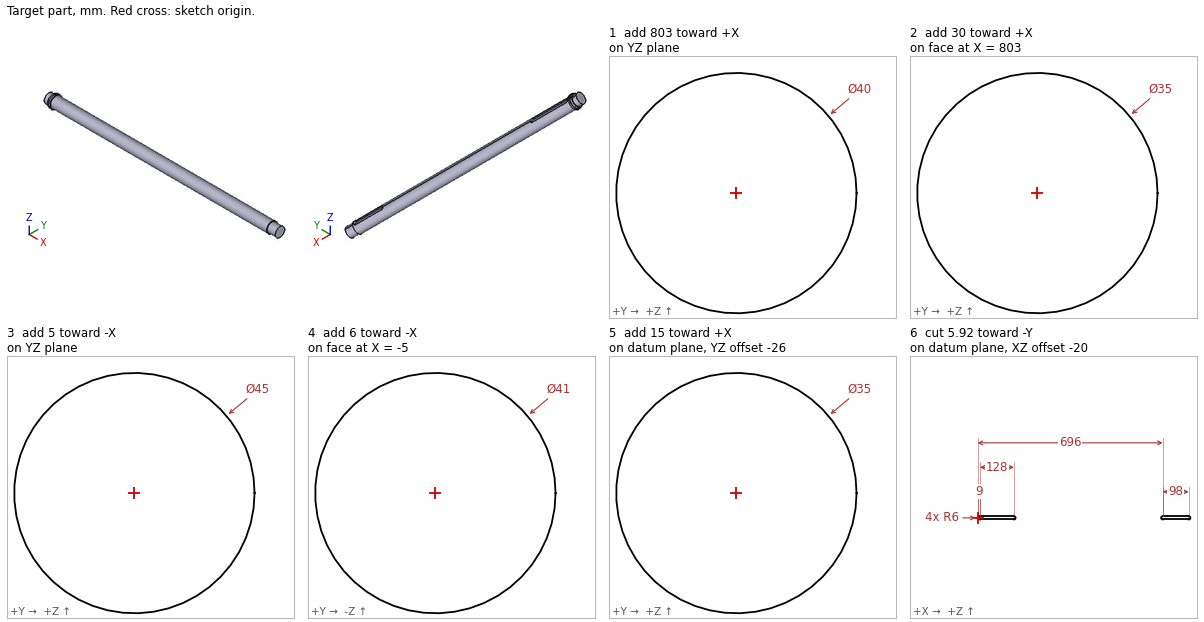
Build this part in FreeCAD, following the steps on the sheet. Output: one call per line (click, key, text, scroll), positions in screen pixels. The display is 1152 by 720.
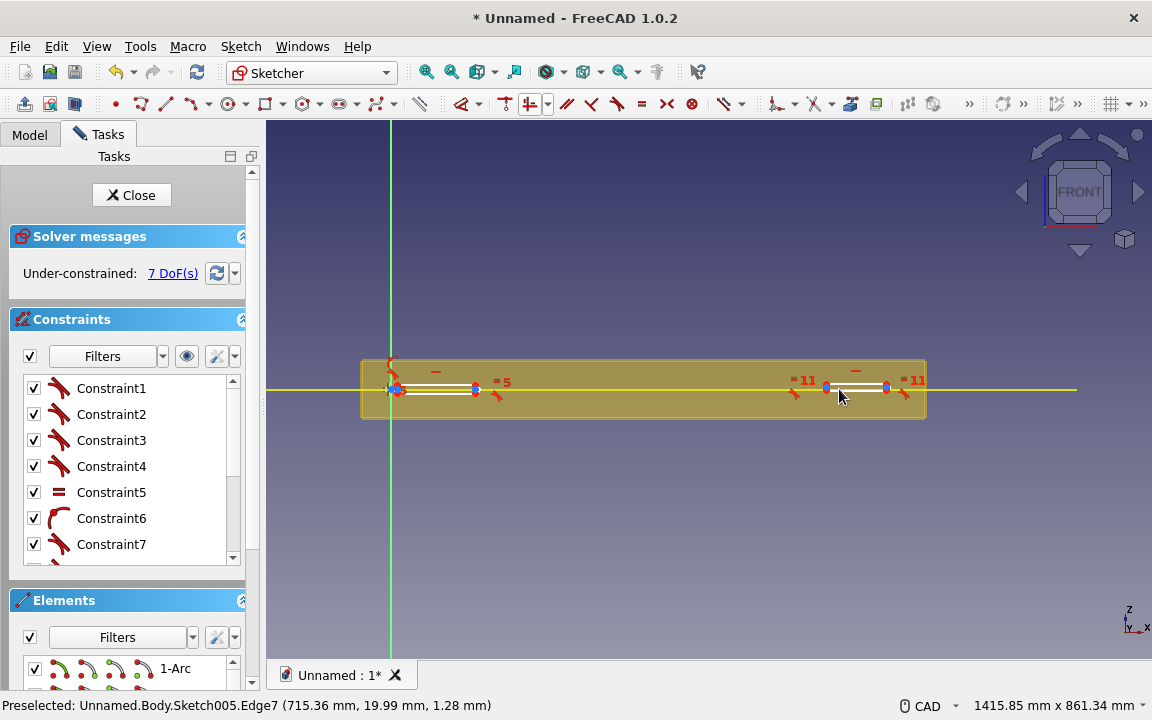
scroll(394, 387, up, 9)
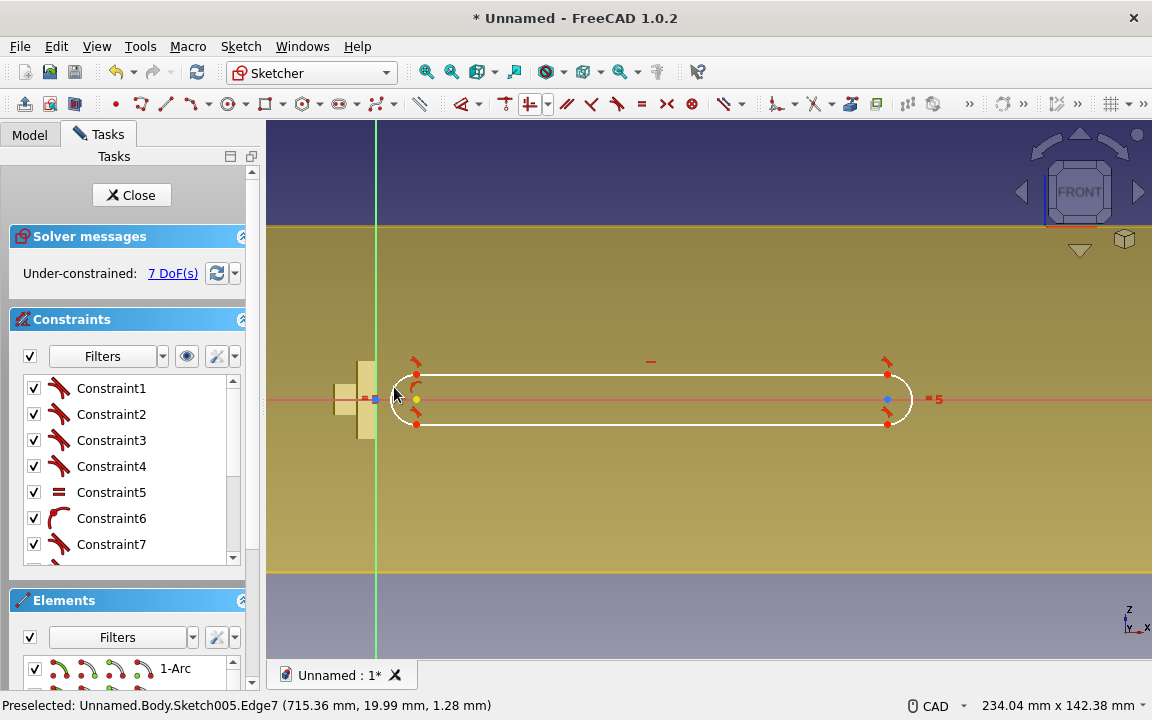
click(396, 385)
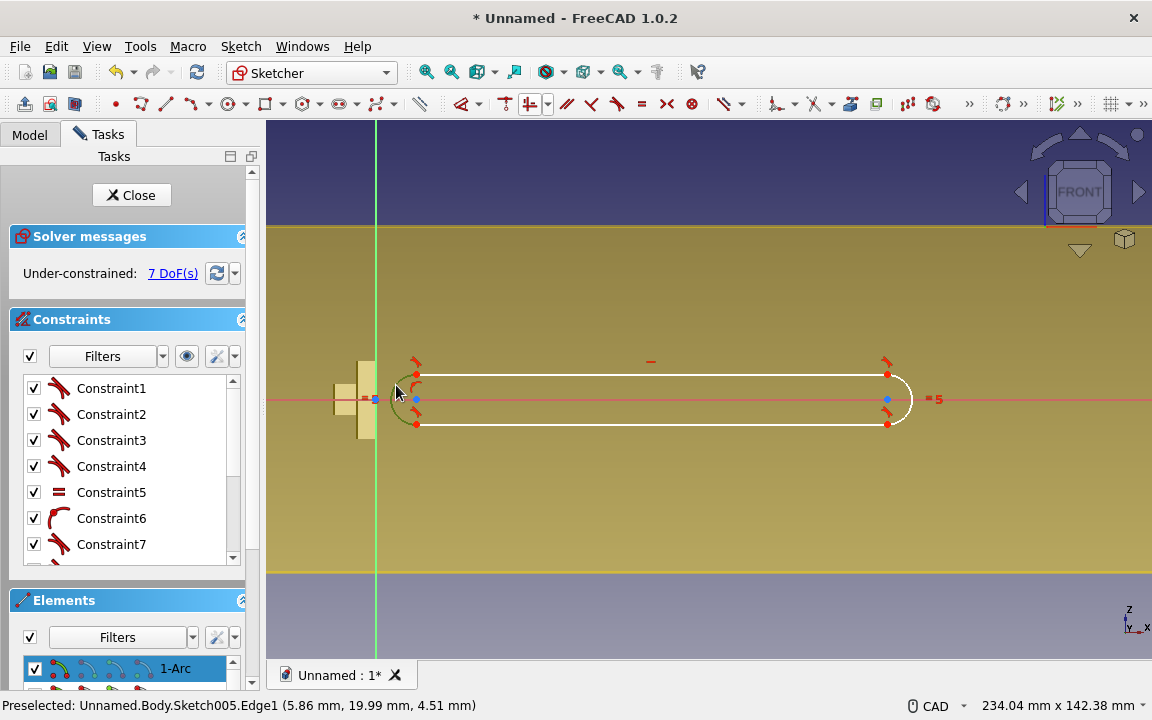
scroll(393, 387, down, 9)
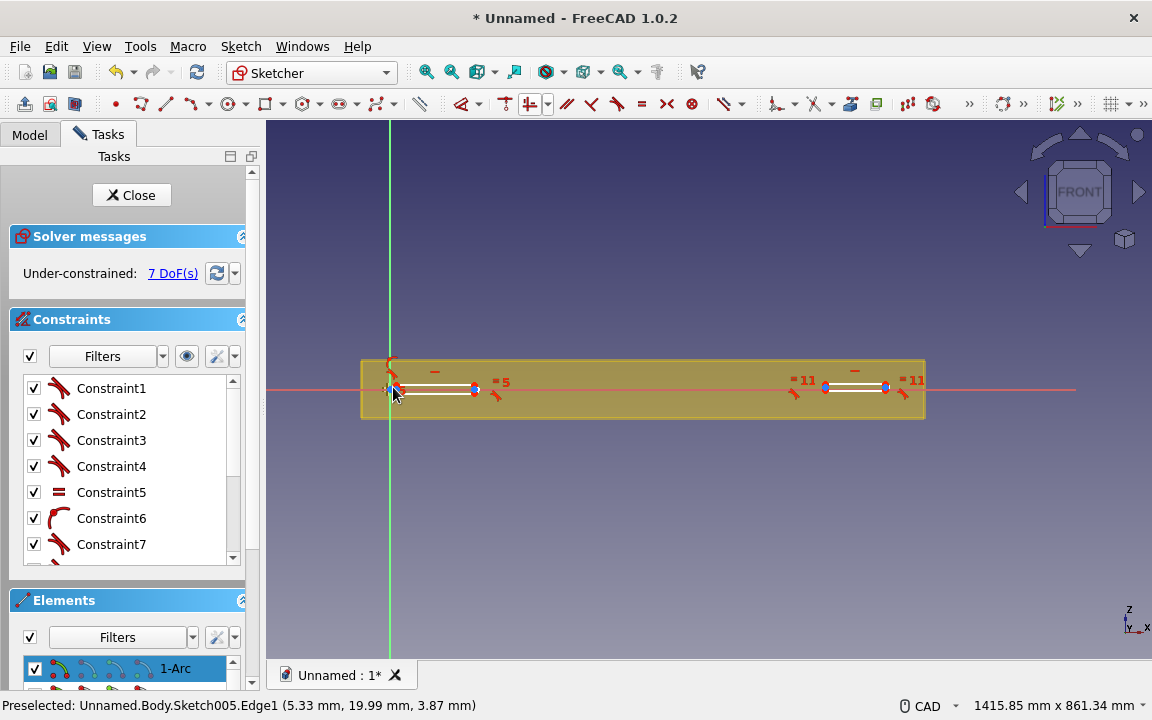
scroll(823, 385, up, 8)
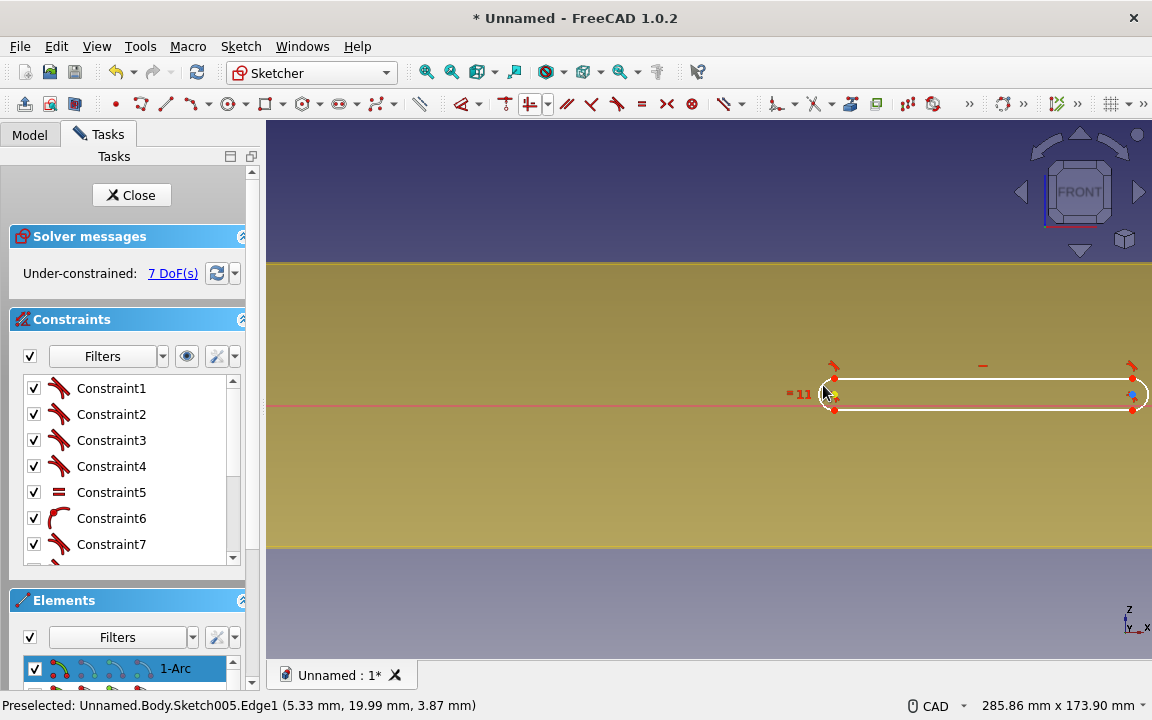
click(822, 385)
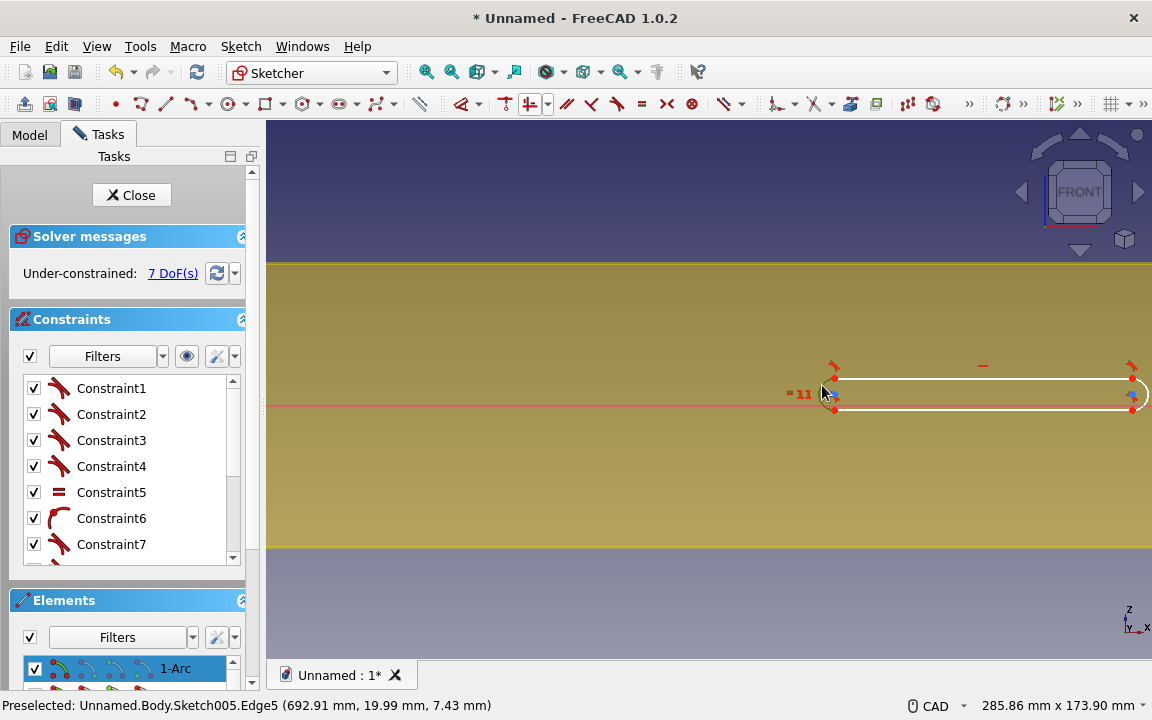
click(642, 104)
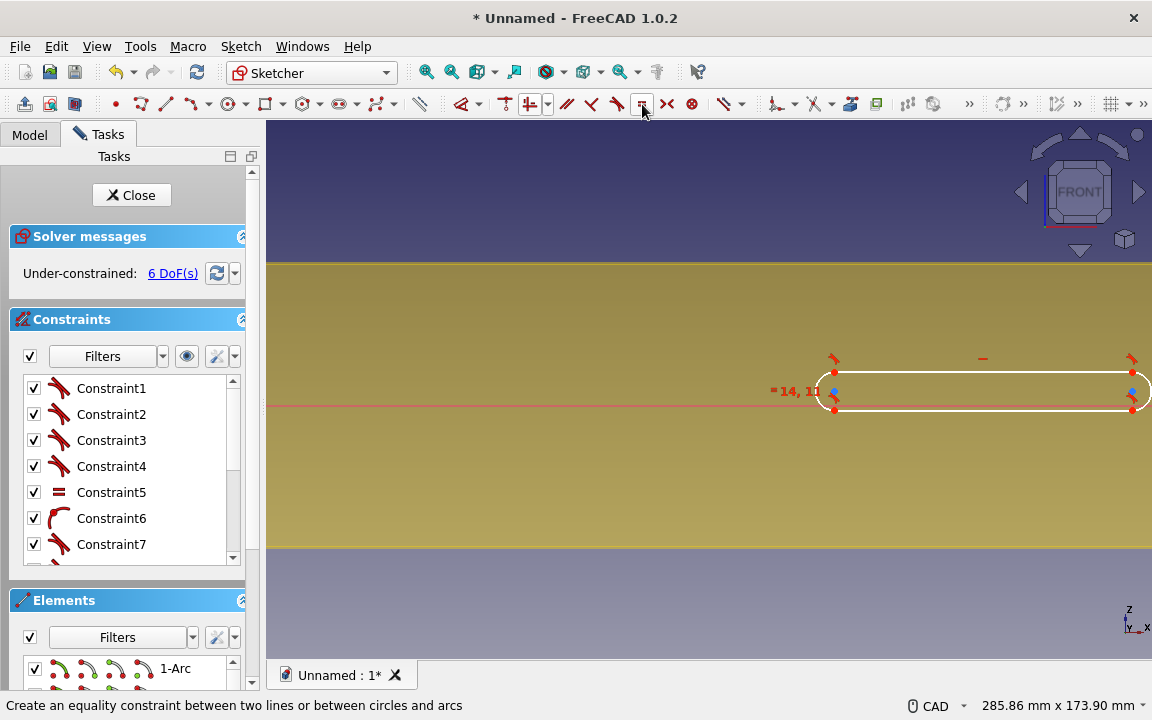
click(835, 391)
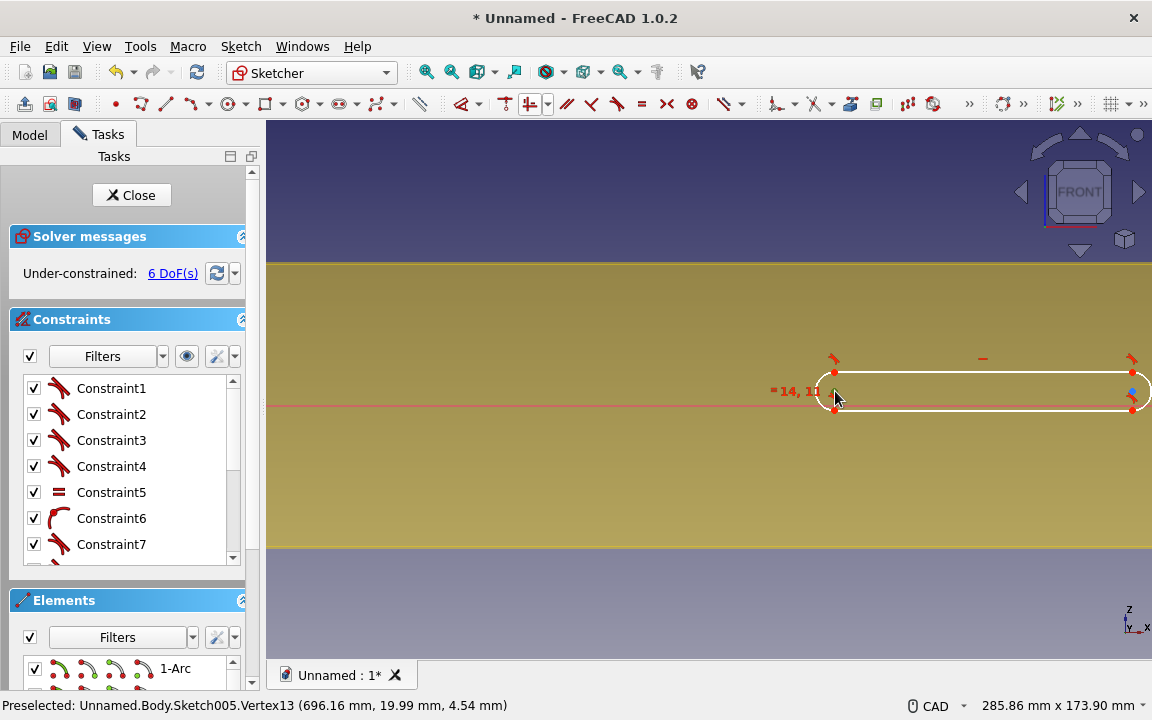
click(344, 406)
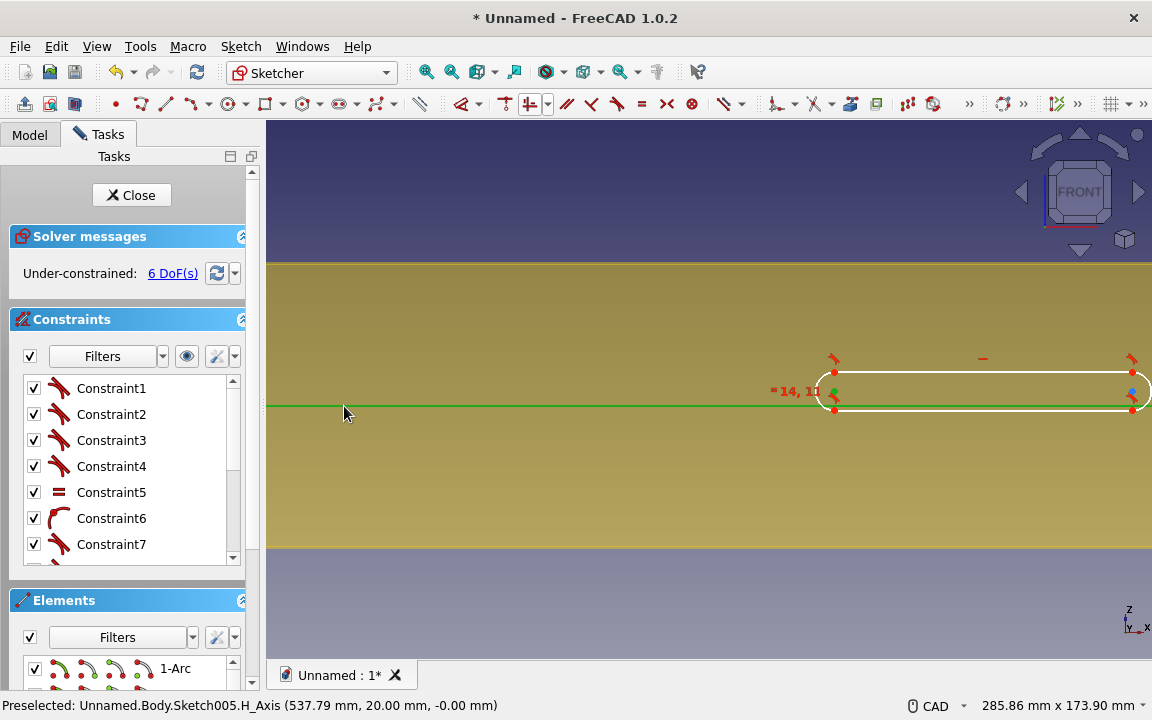
click(505, 104)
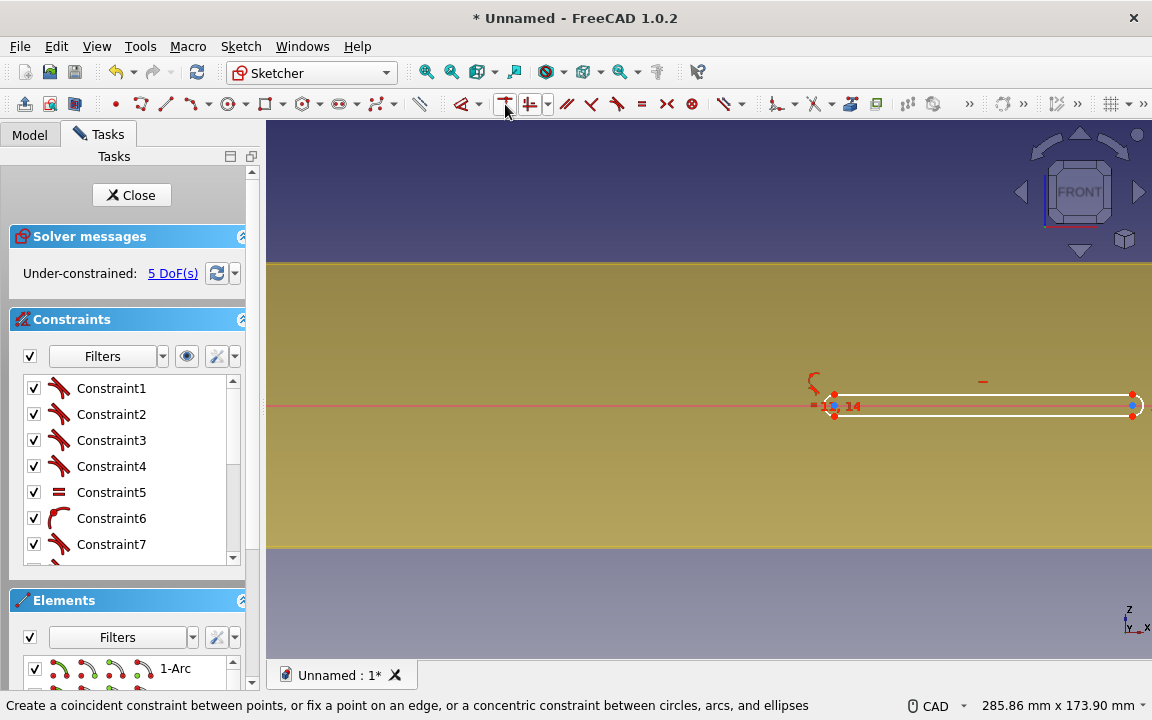
click(460, 104)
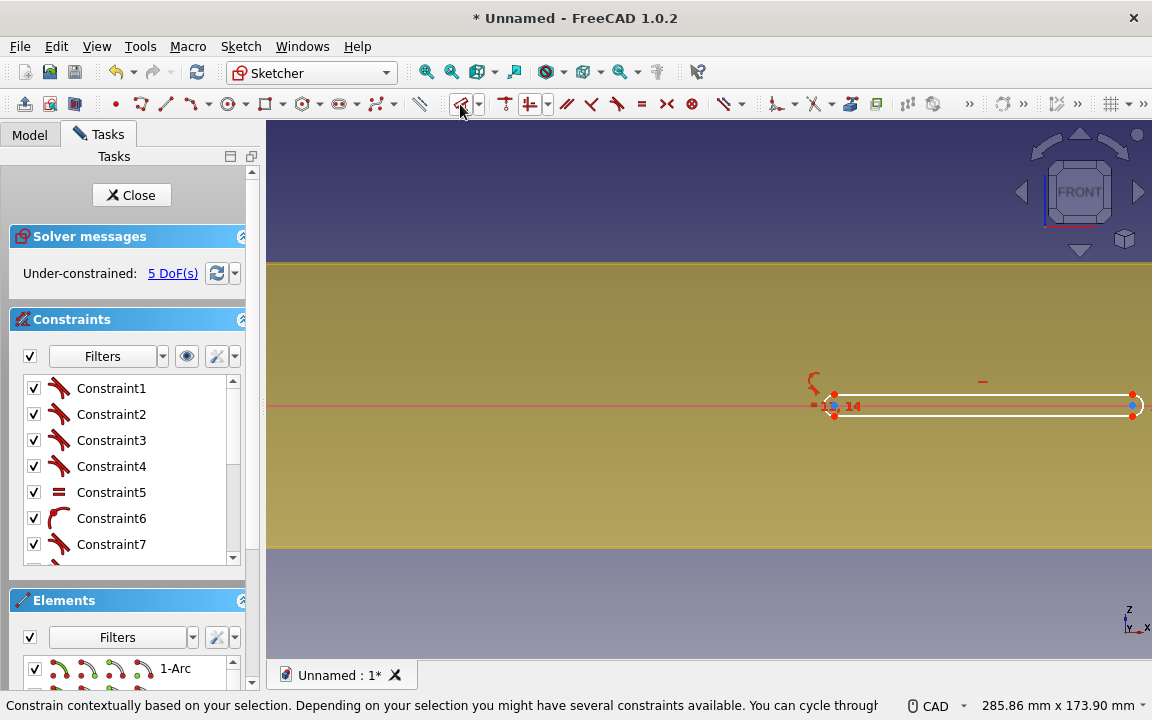
scroll(824, 385, down, 8)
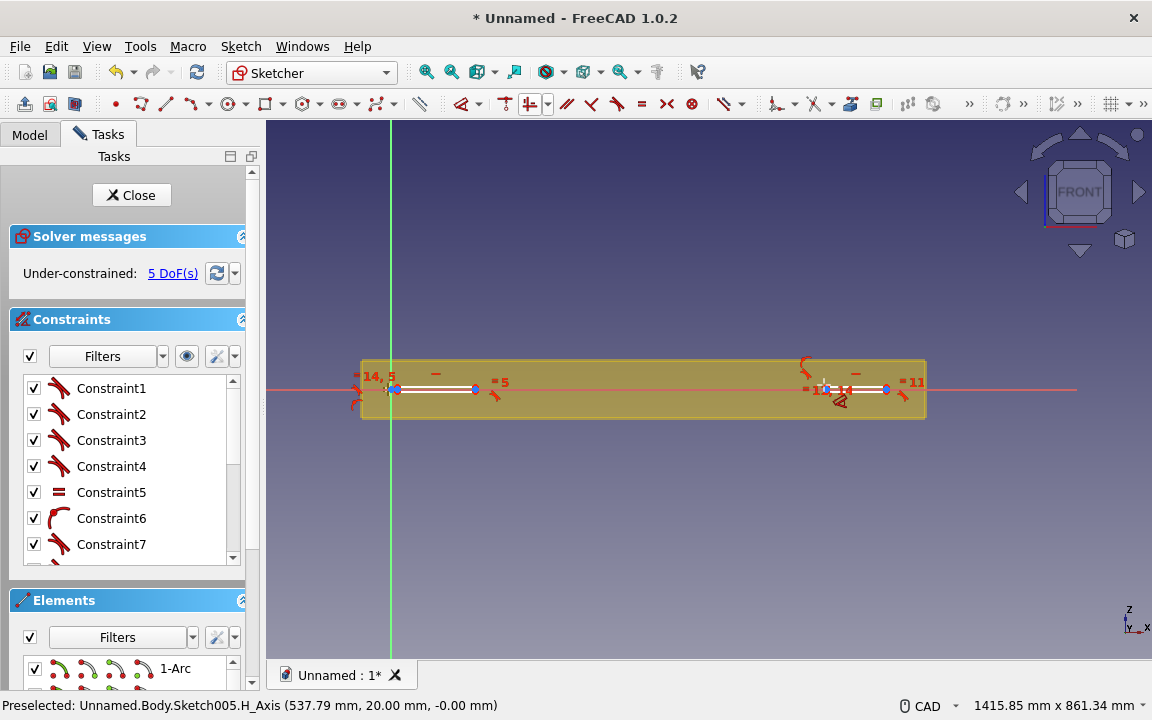
scroll(396, 390, up, 12)